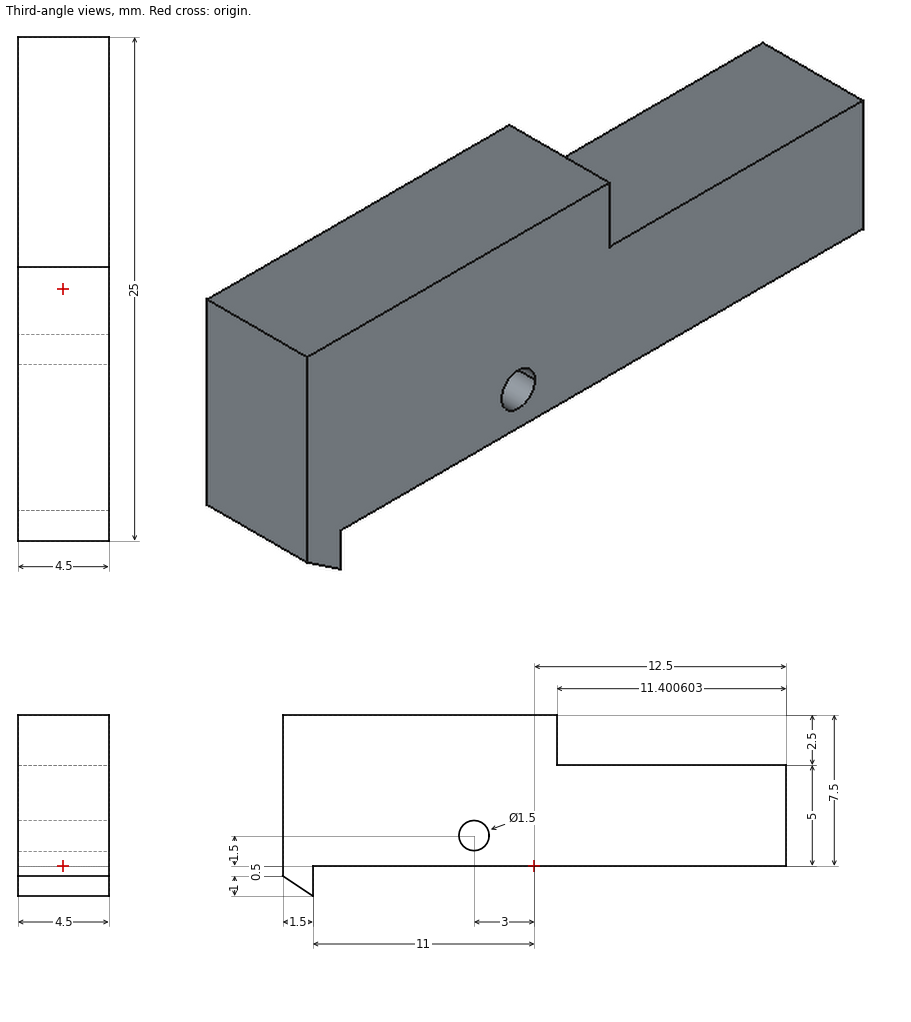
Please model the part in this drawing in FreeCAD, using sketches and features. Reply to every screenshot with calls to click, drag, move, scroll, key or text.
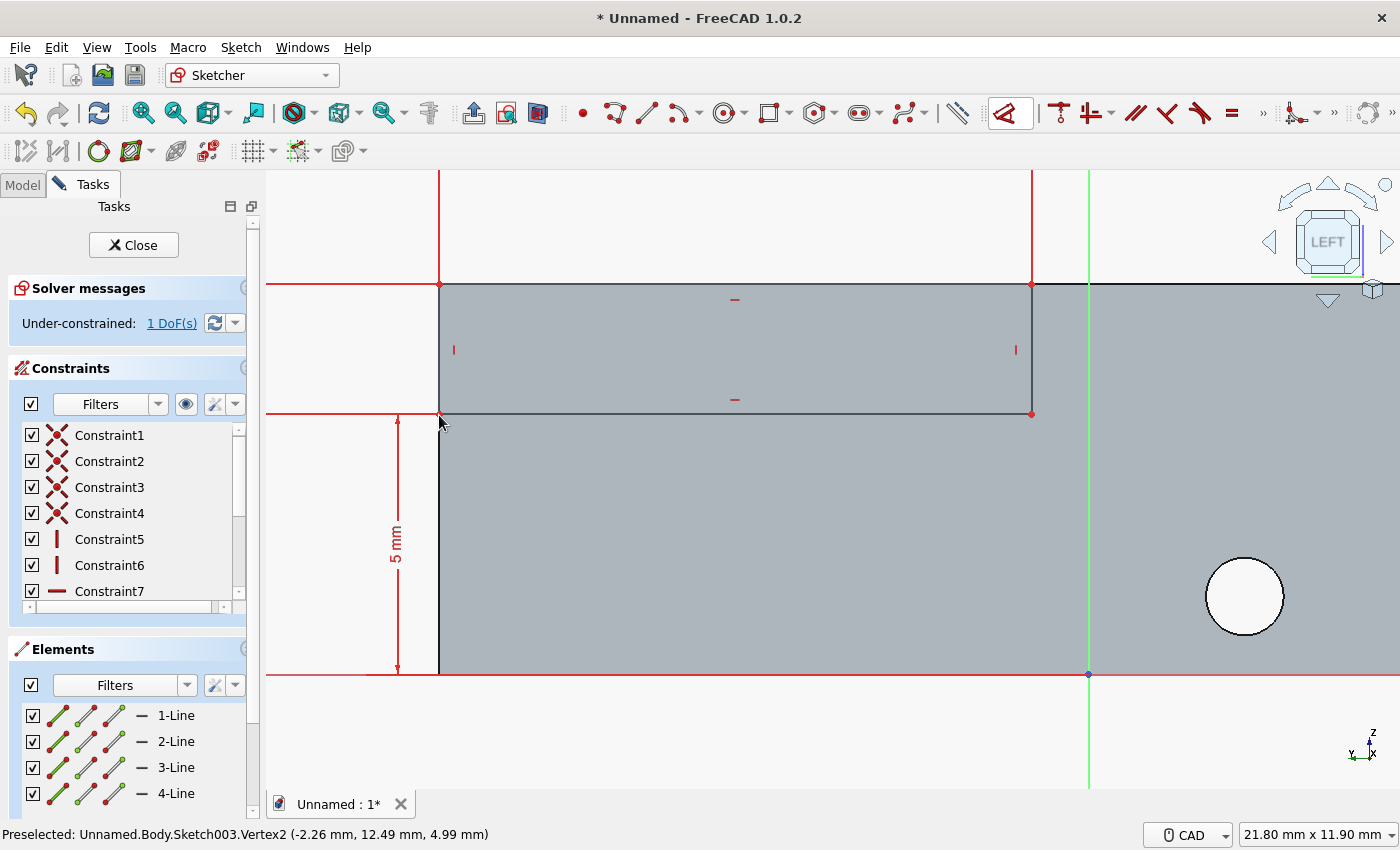
click(439, 284)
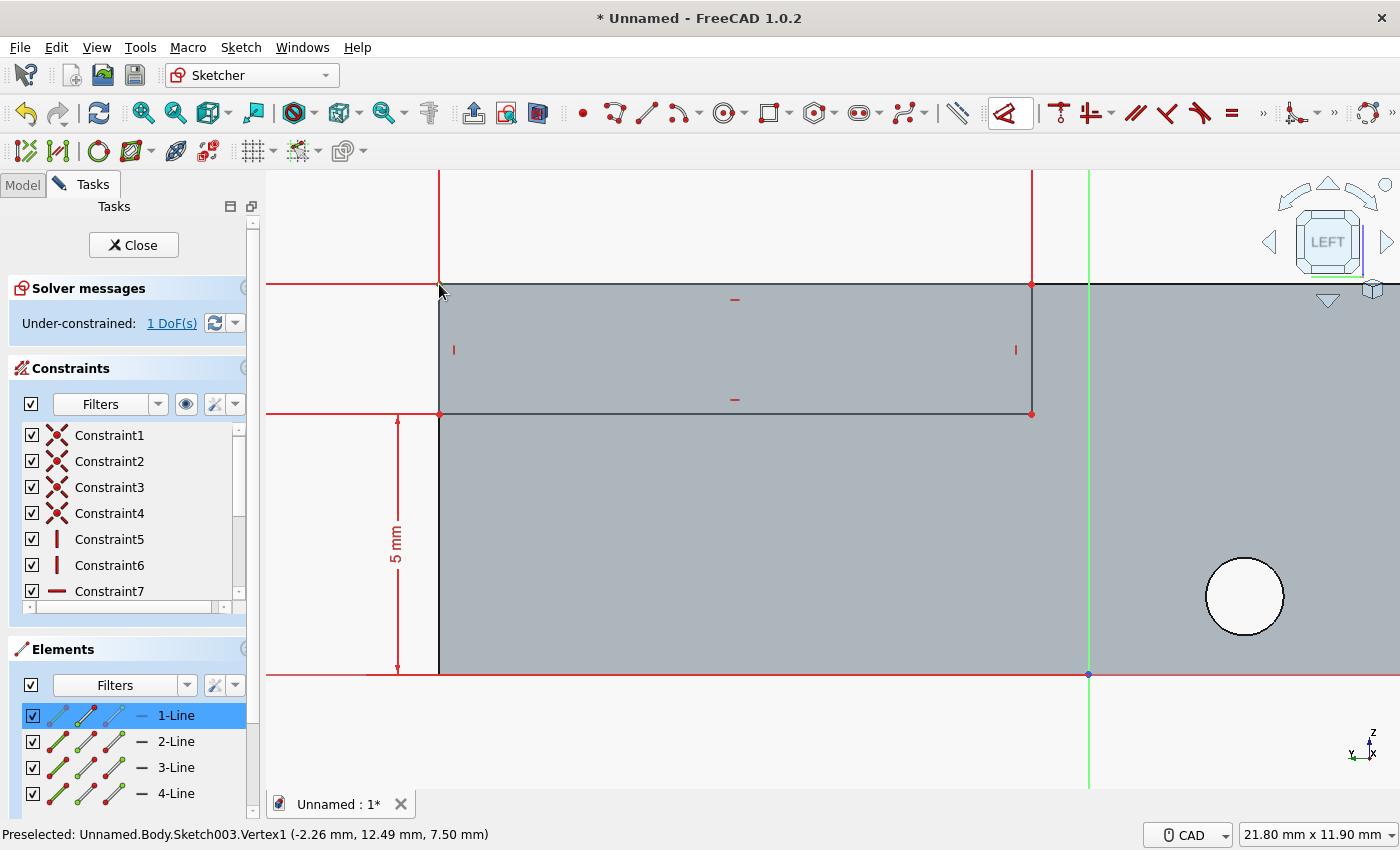
key(l)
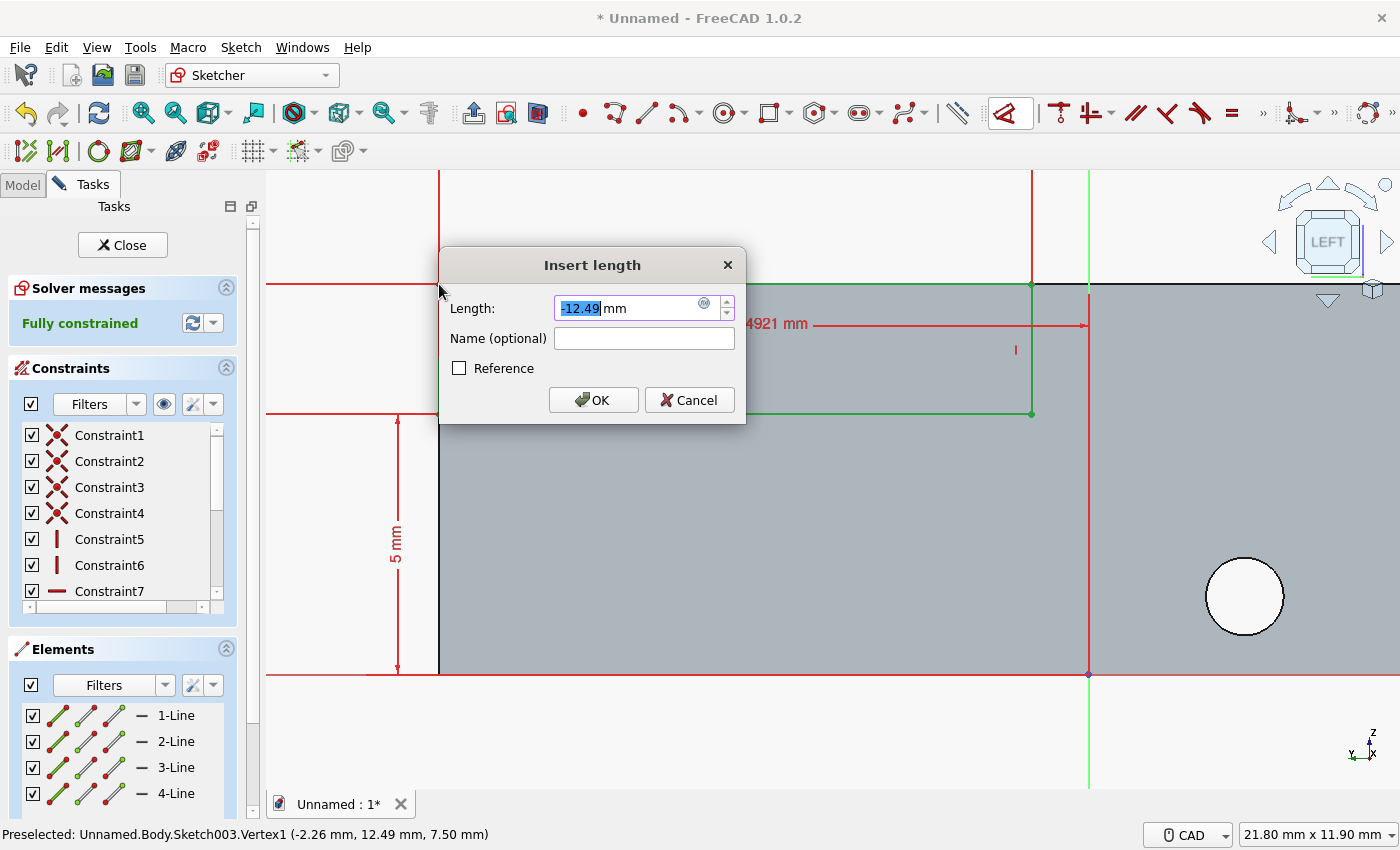
text(-12.5)
key(Return)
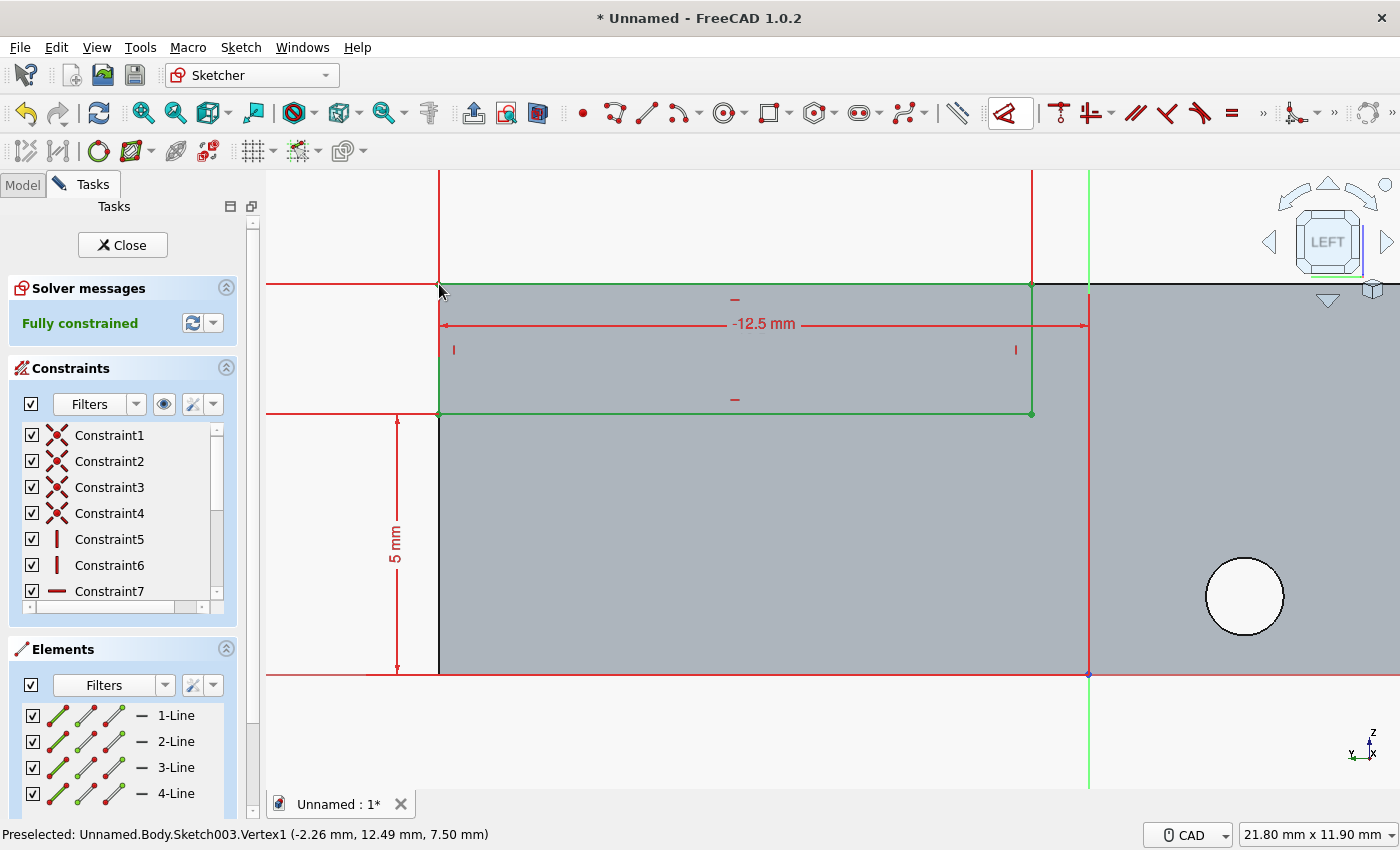
click(123, 245)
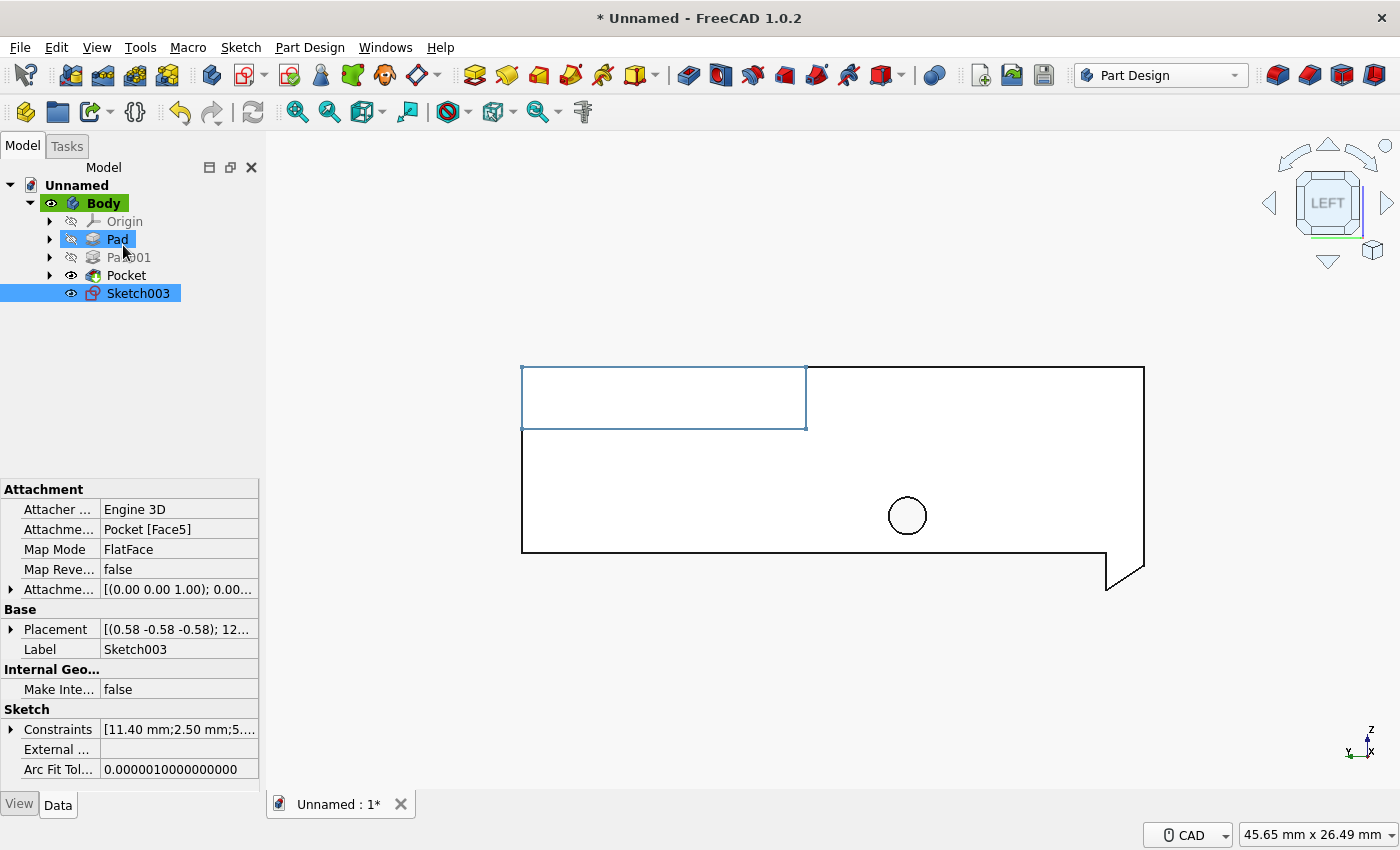
click(690, 76)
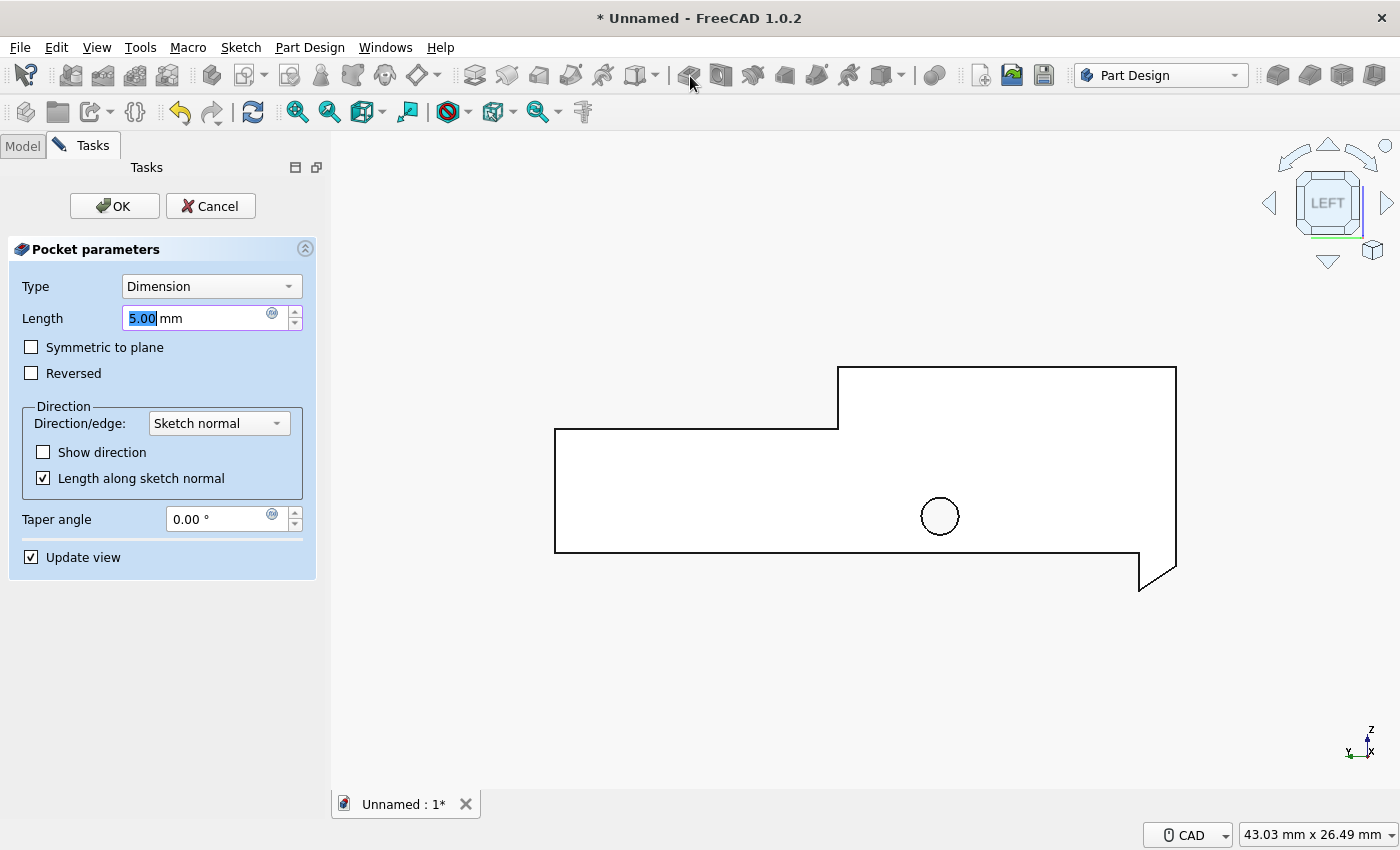
click(212, 286)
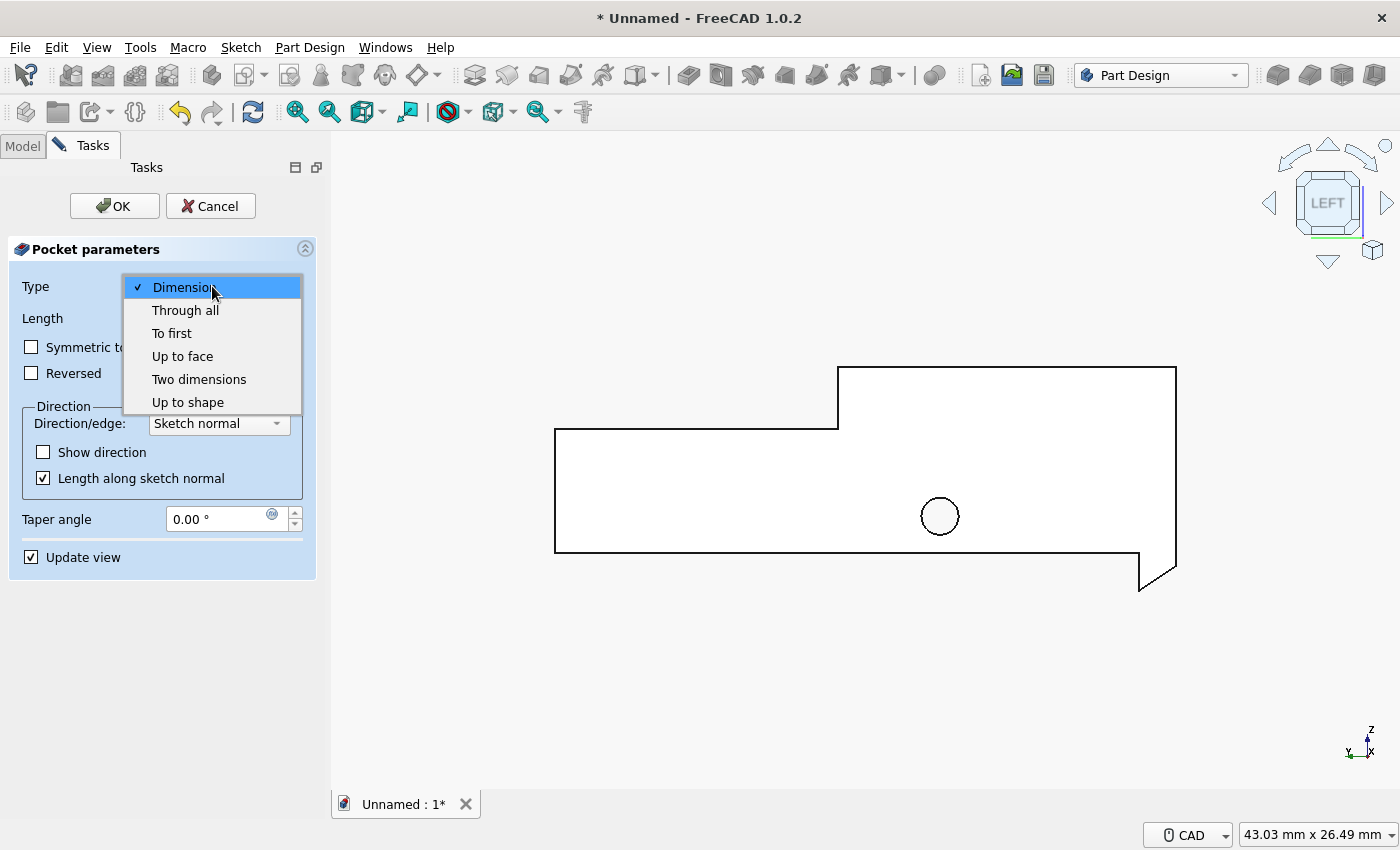
click(212, 310)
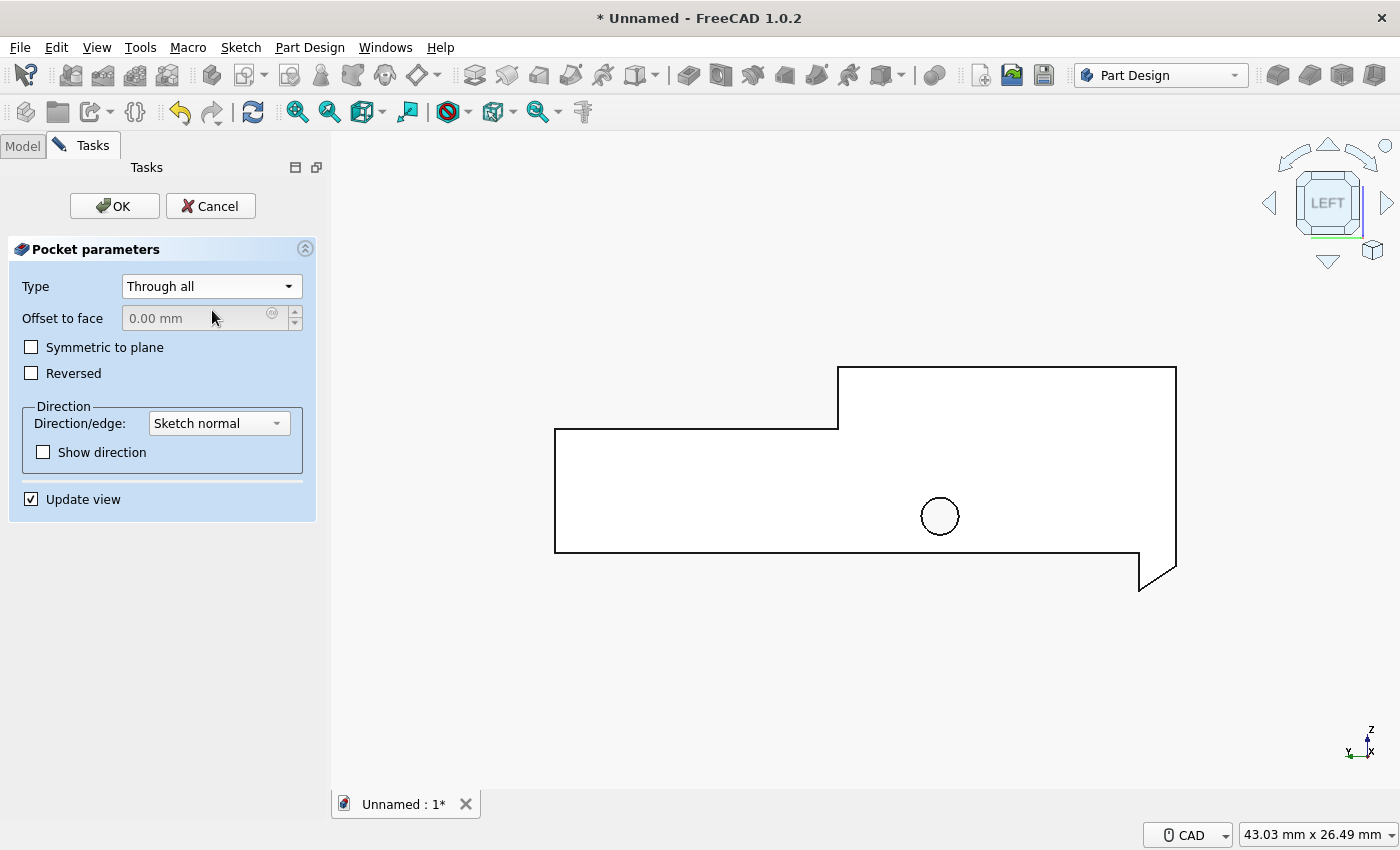
click(115, 206)